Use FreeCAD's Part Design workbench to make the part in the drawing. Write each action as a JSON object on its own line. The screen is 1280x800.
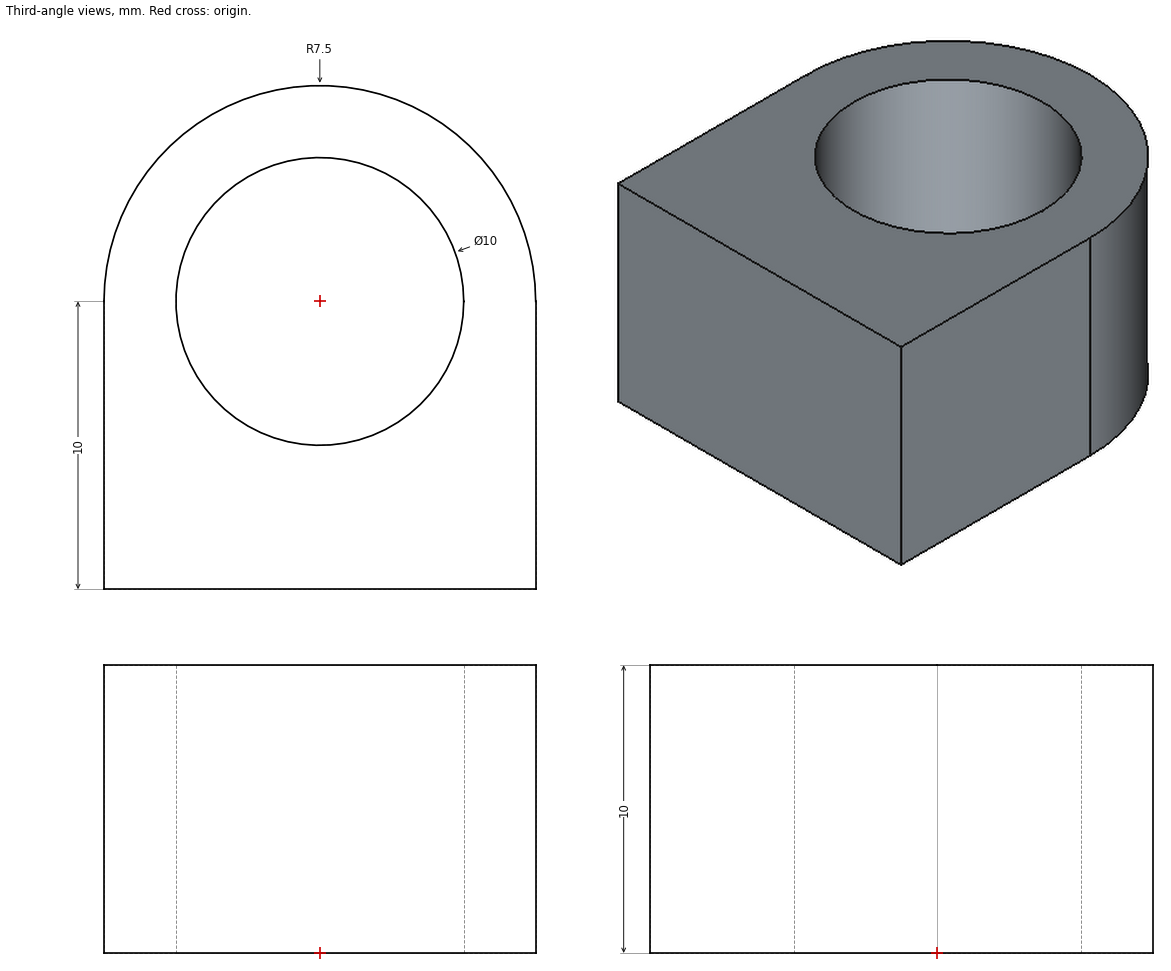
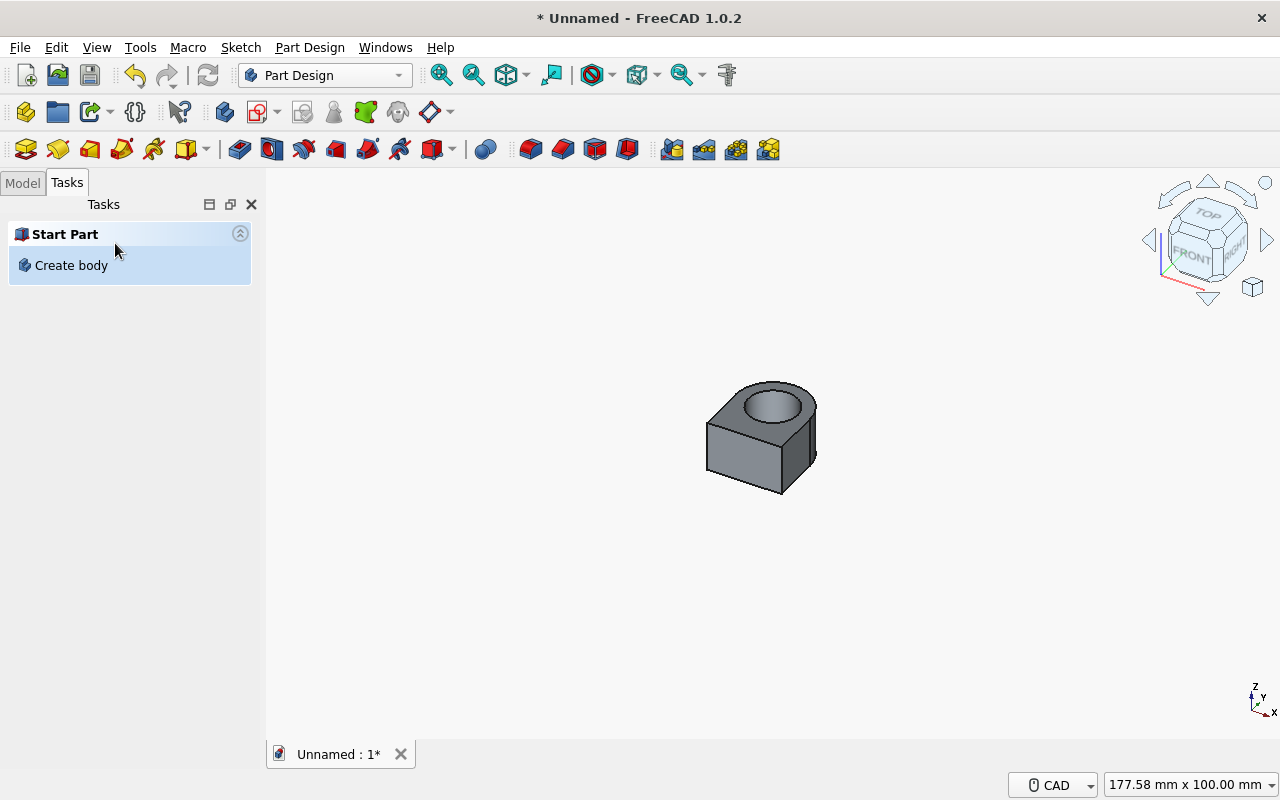
{"action": "key", "text": "0"}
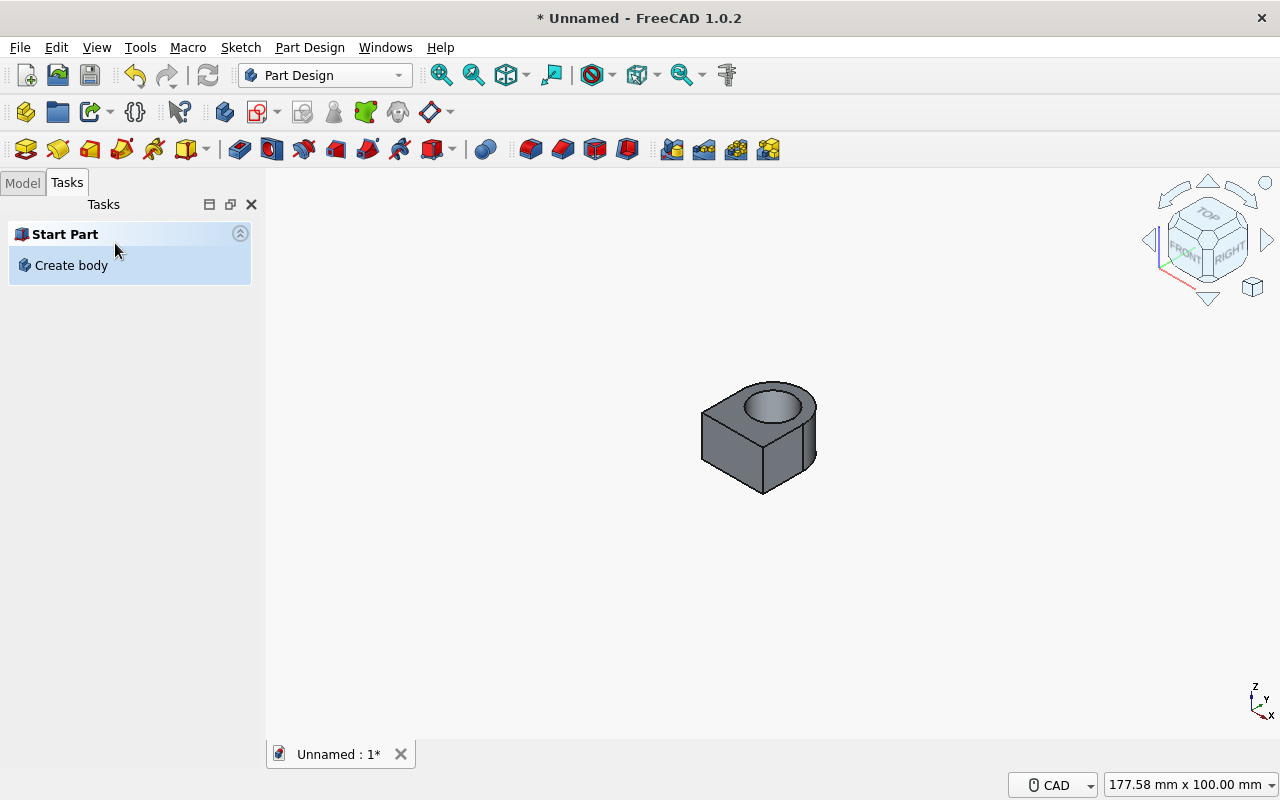
{"action": "left_click", "coordinate": [442, 76]}